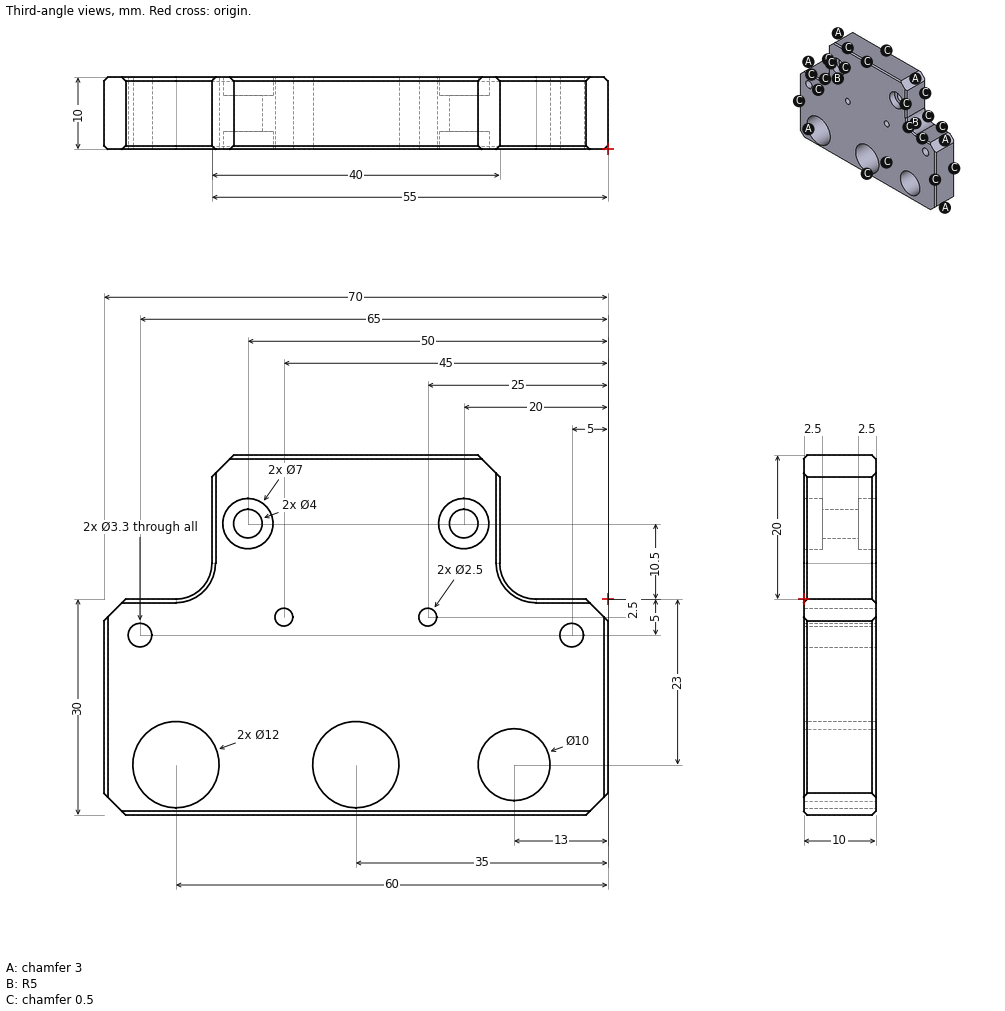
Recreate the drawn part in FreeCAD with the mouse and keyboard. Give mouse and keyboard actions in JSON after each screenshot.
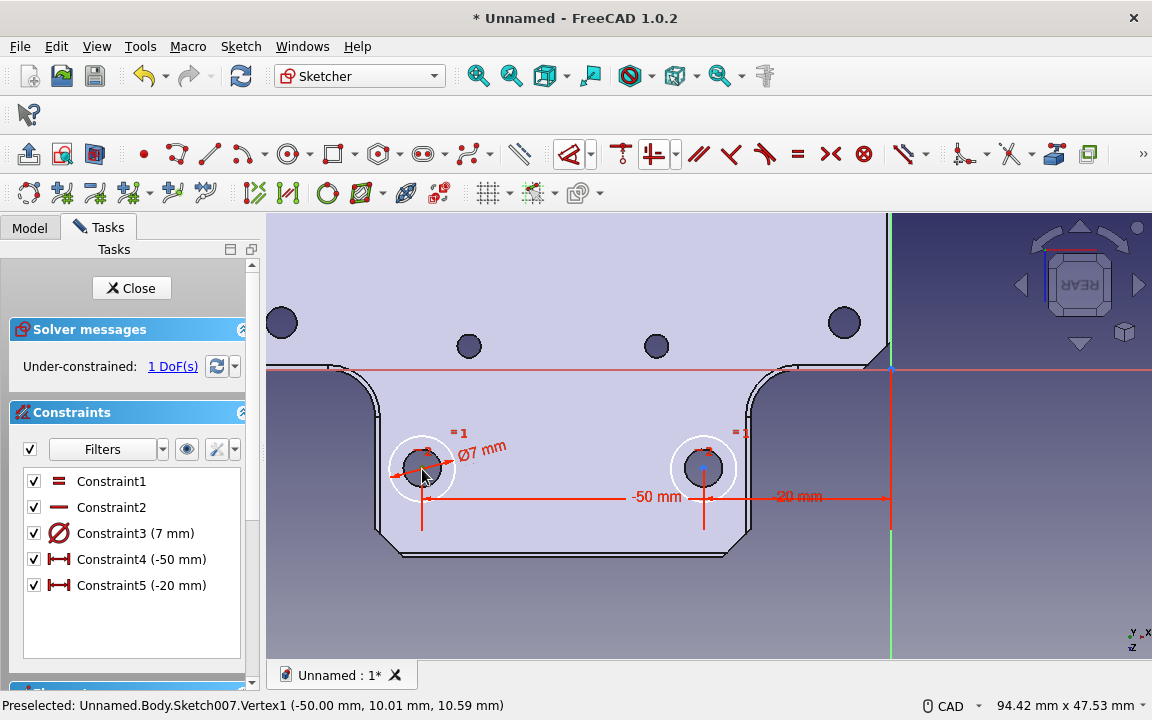
{"action": "left_click", "coordinate": [590, 154]}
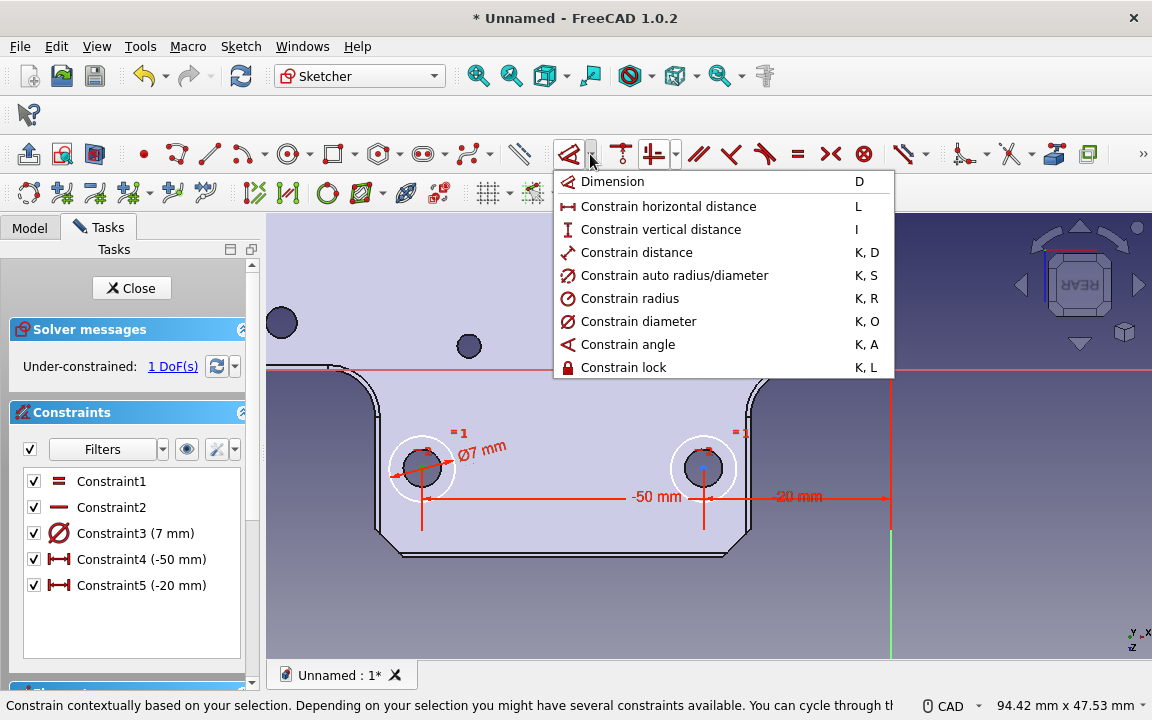
{"action": "left_click", "coordinate": [724, 230]}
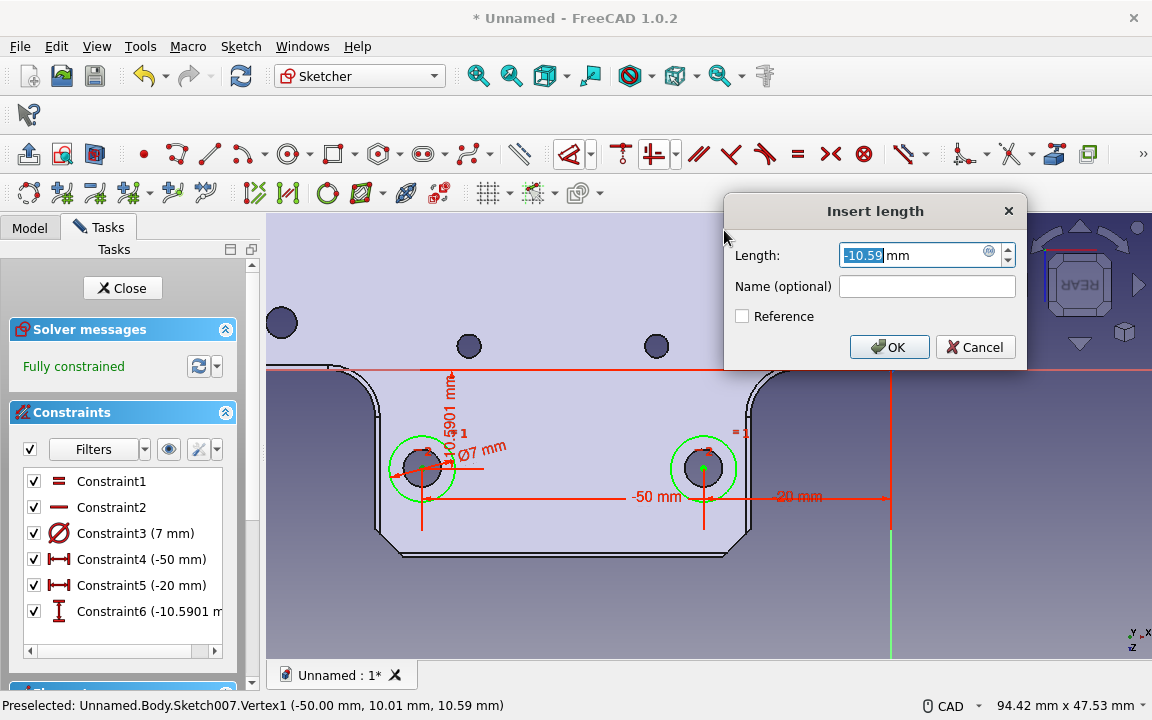
{"action": "type", "text": "-10.5"}
{"action": "key", "text": "Return"}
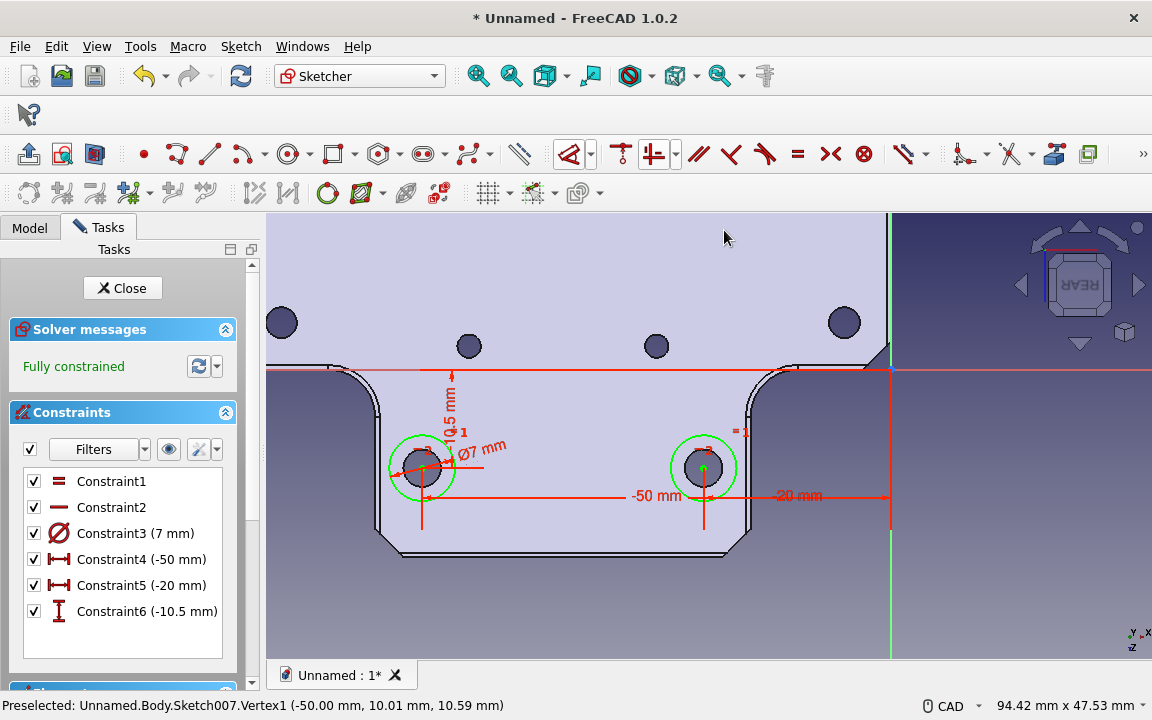
{"action": "left_click", "coordinate": [123, 288]}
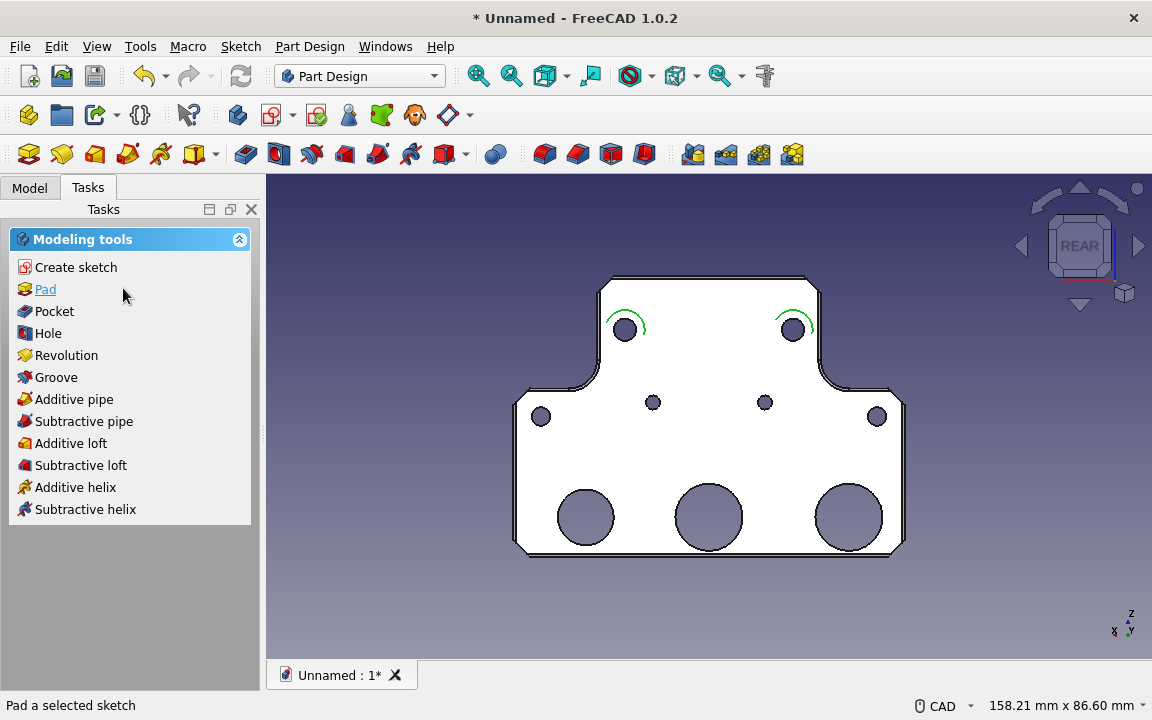
{"action": "left_click", "coordinate": [246, 154]}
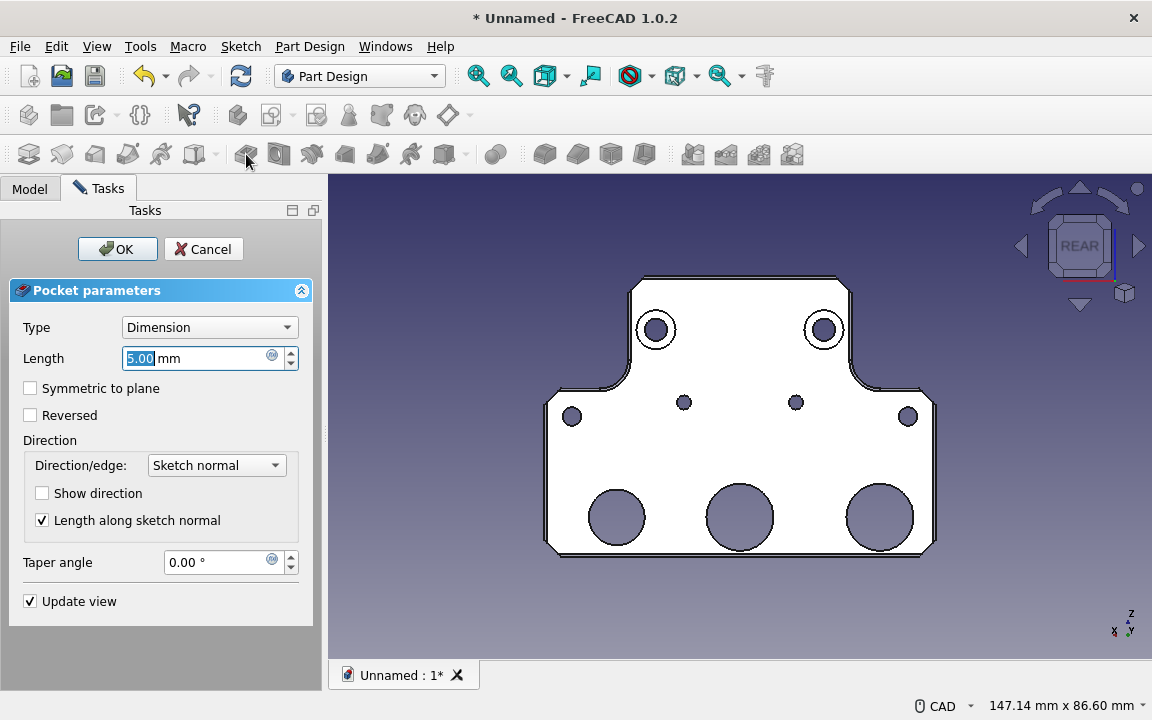
{"action": "type", "text": "2.5"}
{"action": "key", "text": "Tab"}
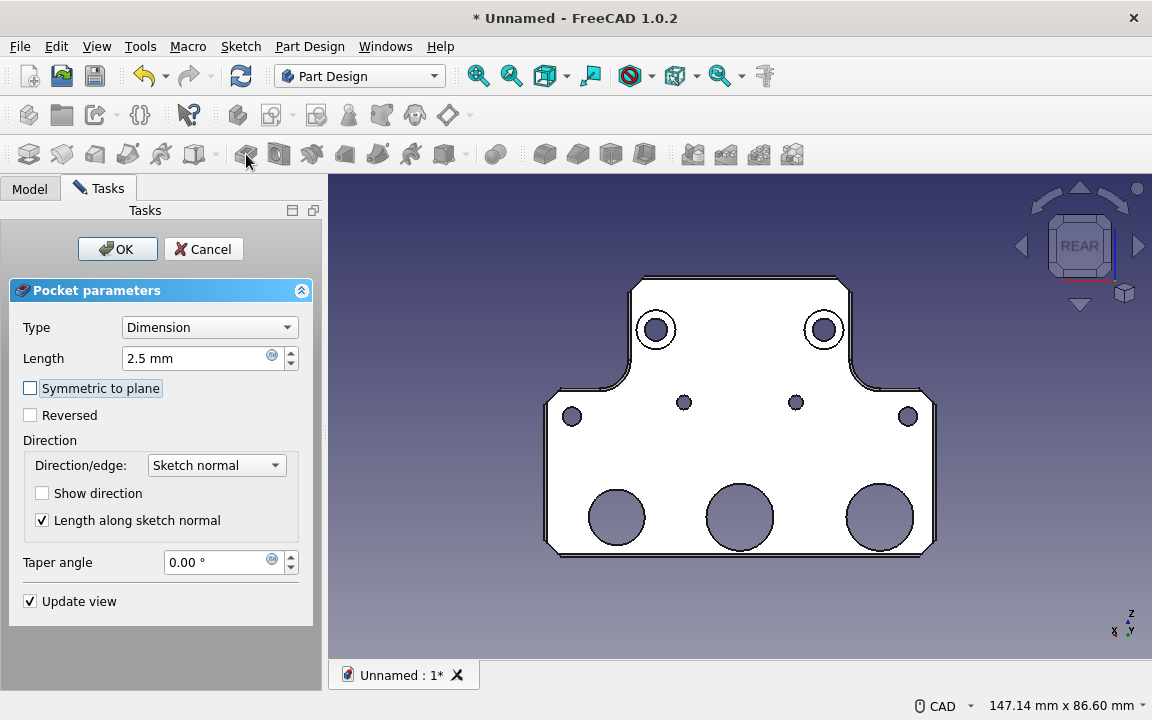
{"action": "left_click", "coordinate": [118, 249]}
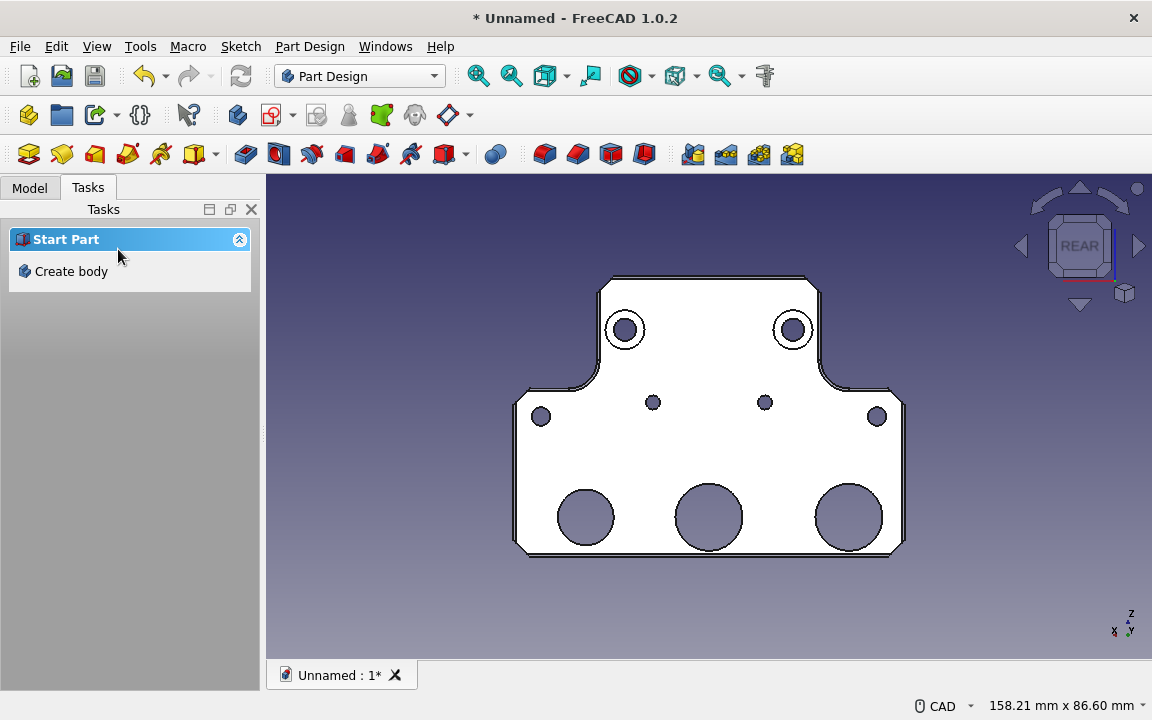
{"action": "left_click", "coordinate": [30, 188]}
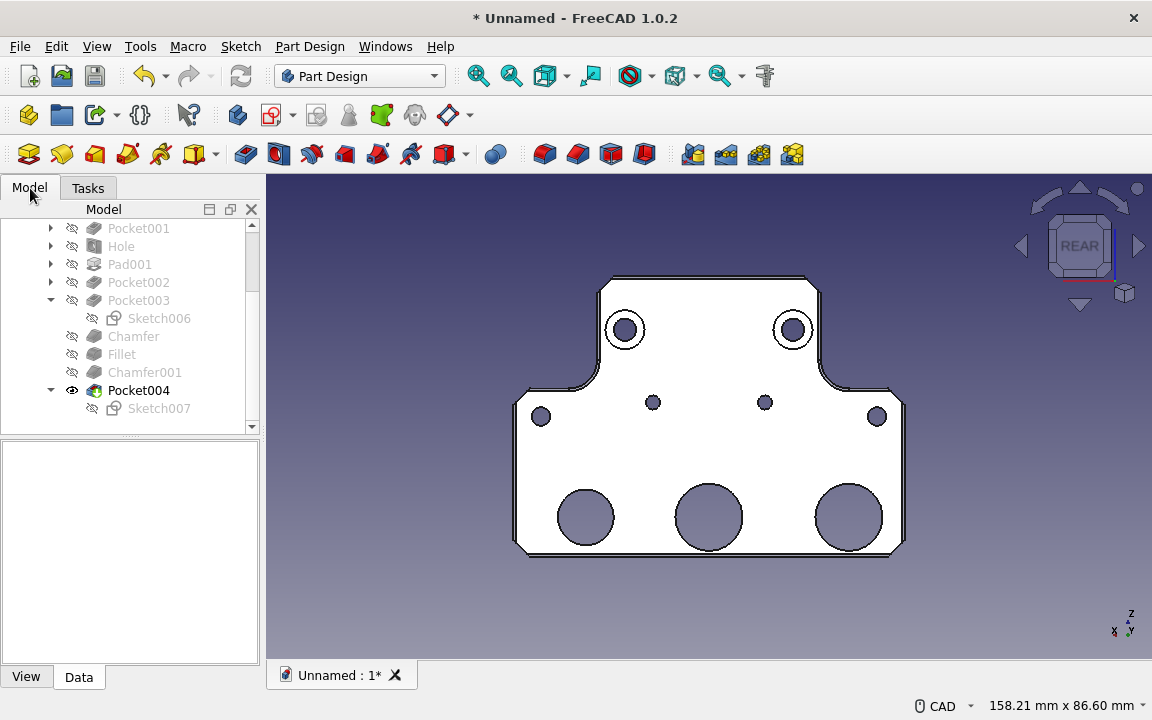
{"action": "scroll", "coordinate": [141, 314], "scroll_direction": "down", "scroll_amount": 3}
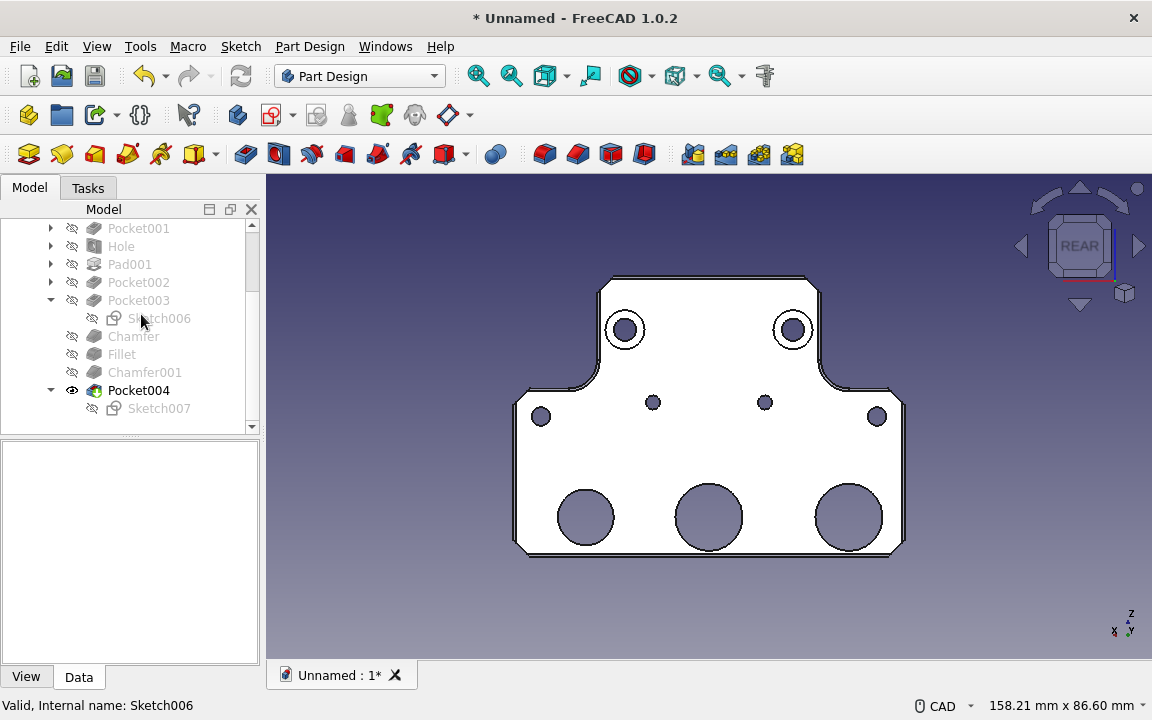
{"action": "scroll", "coordinate": [141, 314], "scroll_direction": "up", "scroll_amount": 15}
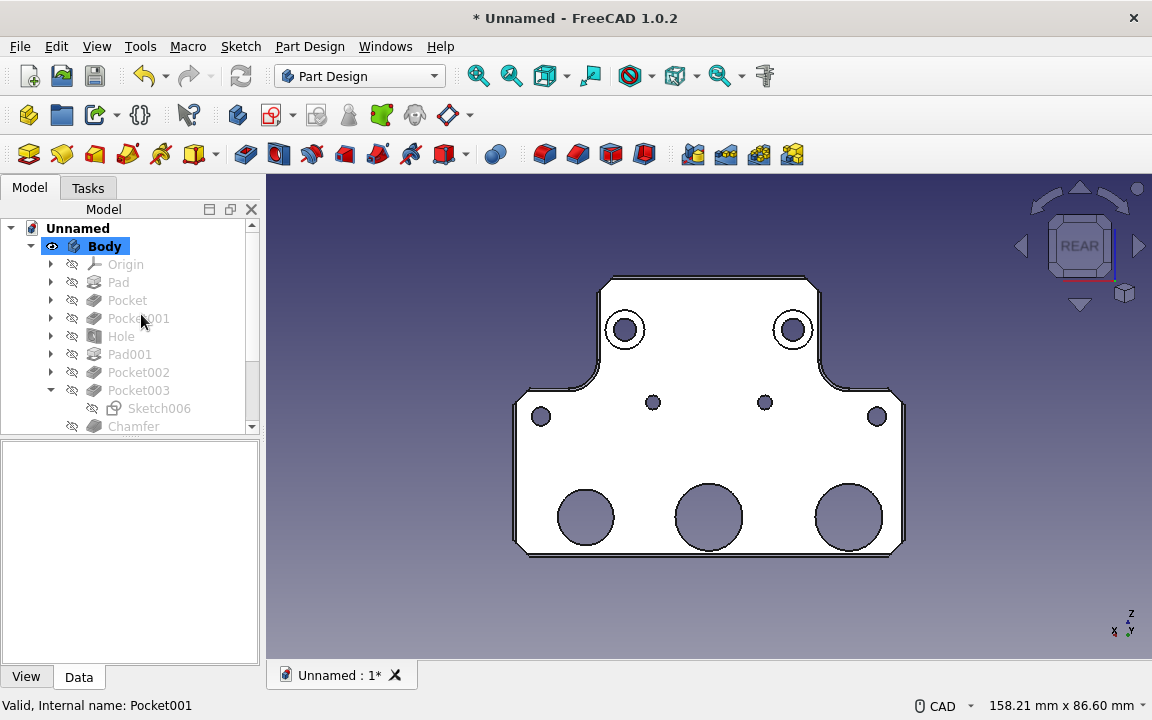
{"action": "left_click", "coordinate": [51, 264]}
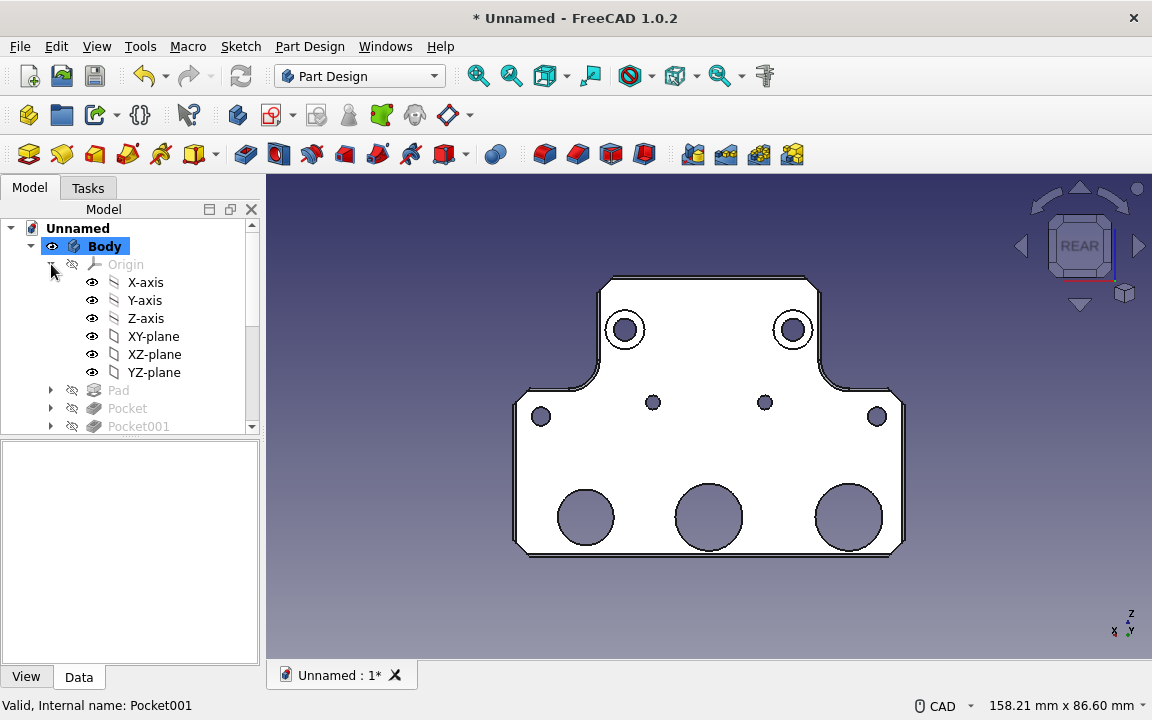
{"action": "left_click", "coordinate": [137, 354]}